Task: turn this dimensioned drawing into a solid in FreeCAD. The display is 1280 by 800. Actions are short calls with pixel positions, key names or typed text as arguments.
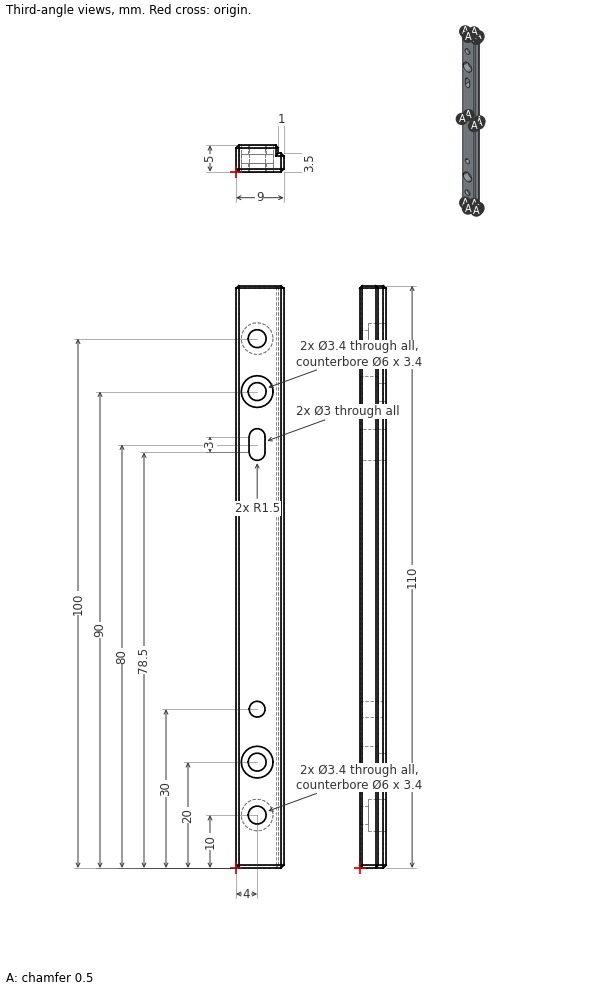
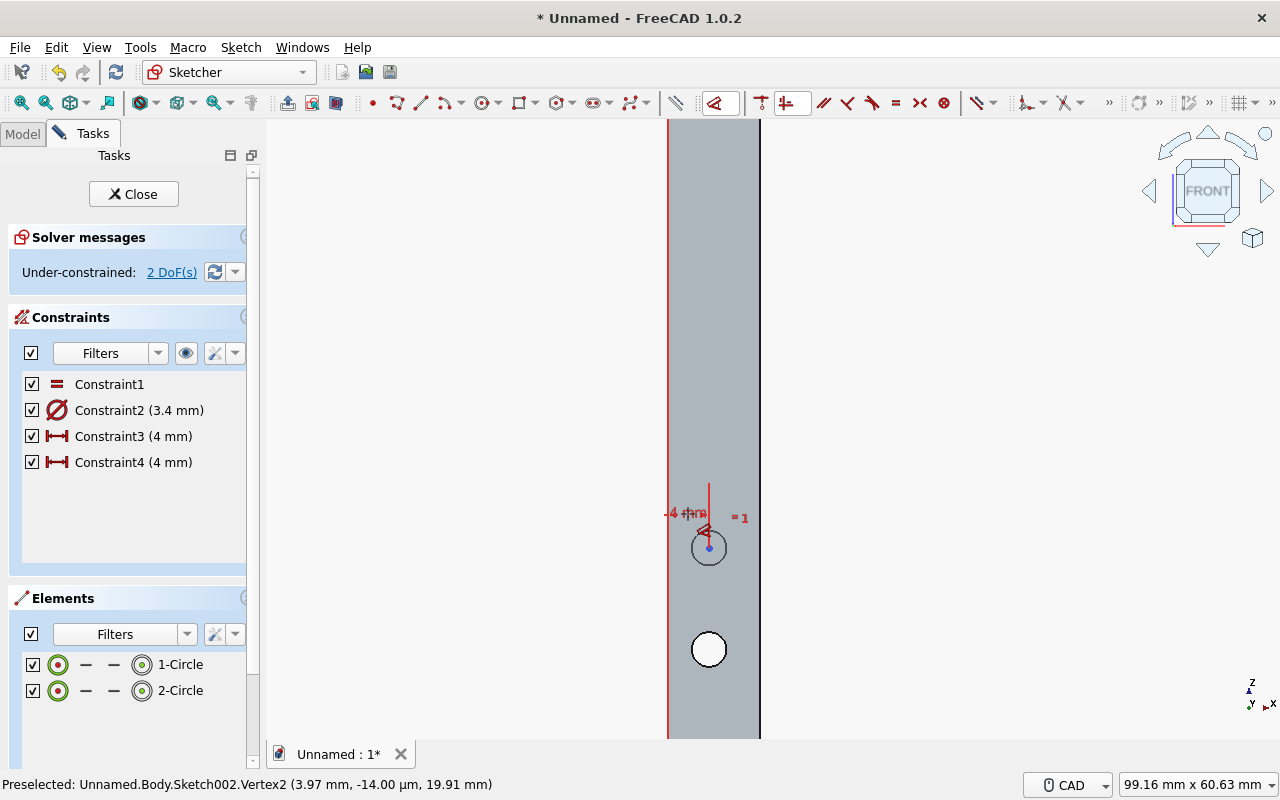
scroll(710, 548, down, 4)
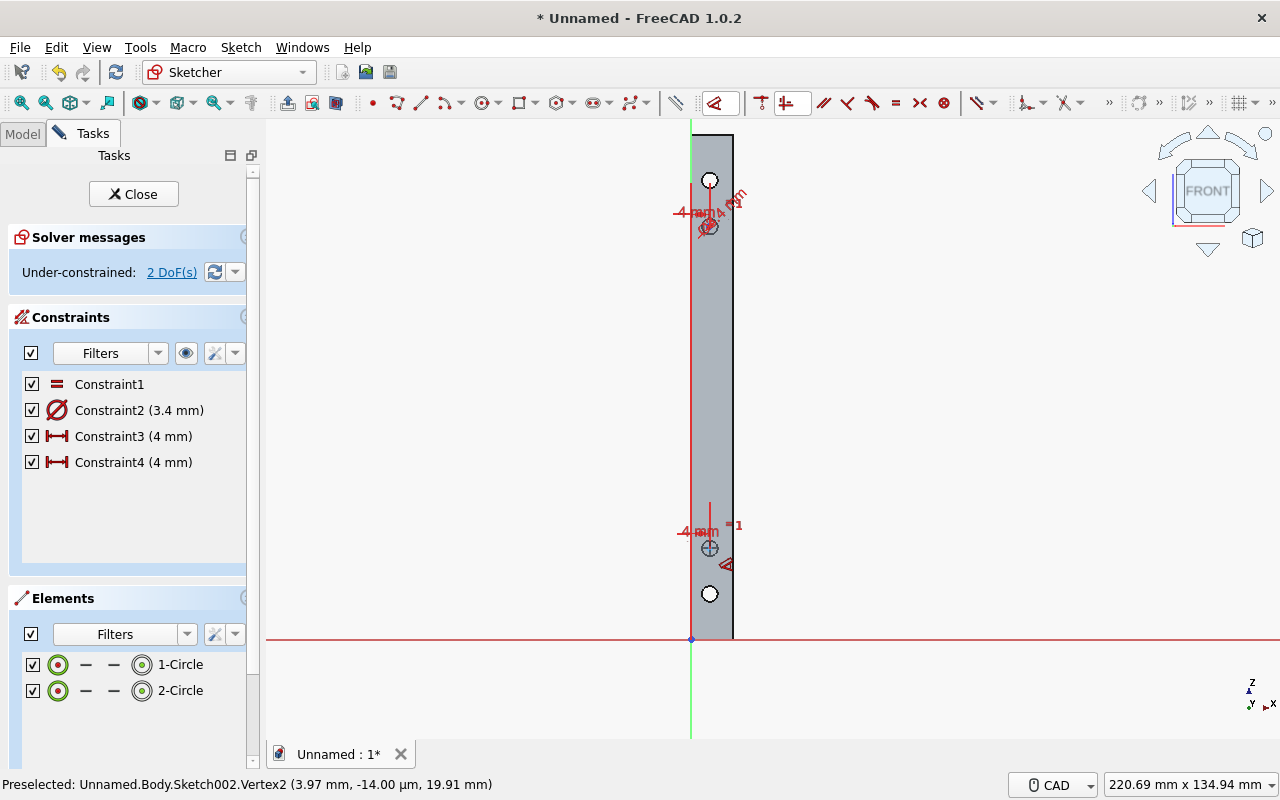
click(710, 227)
click(657, 433)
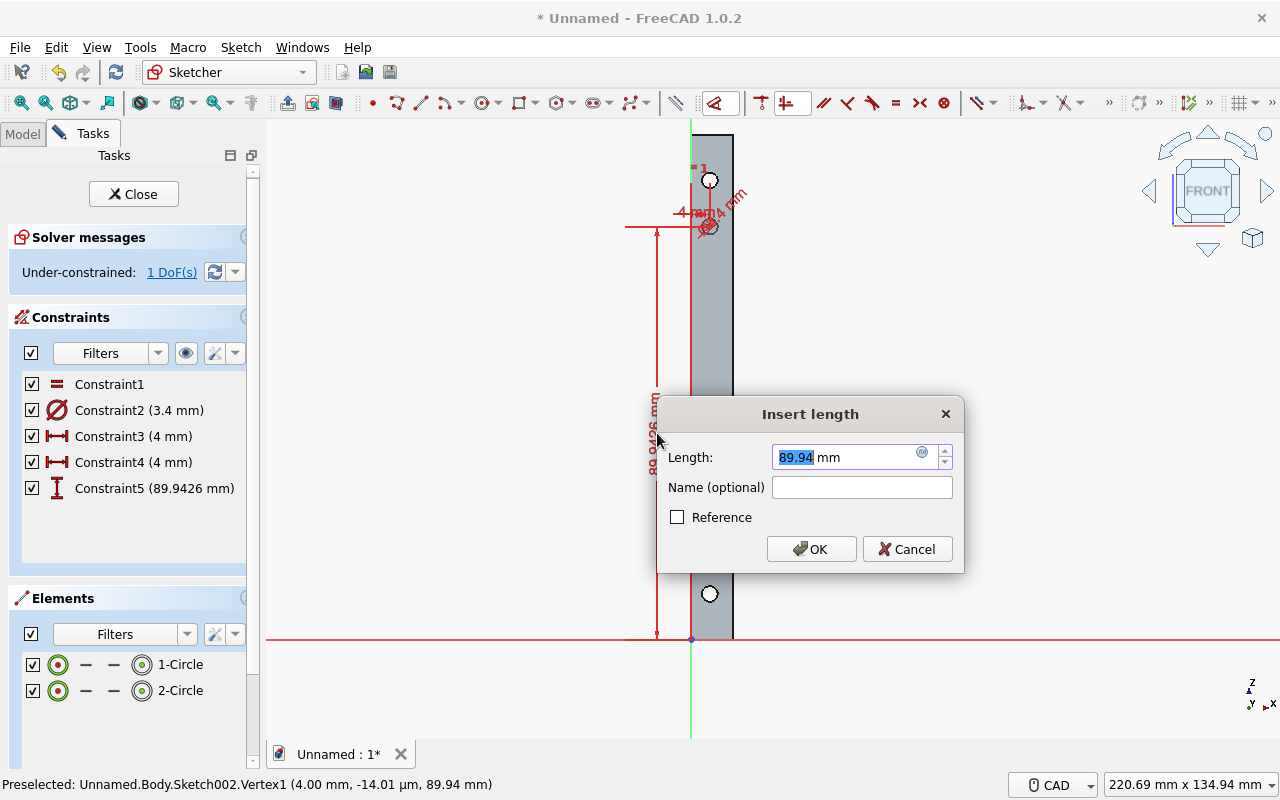
text(90)
key(Return)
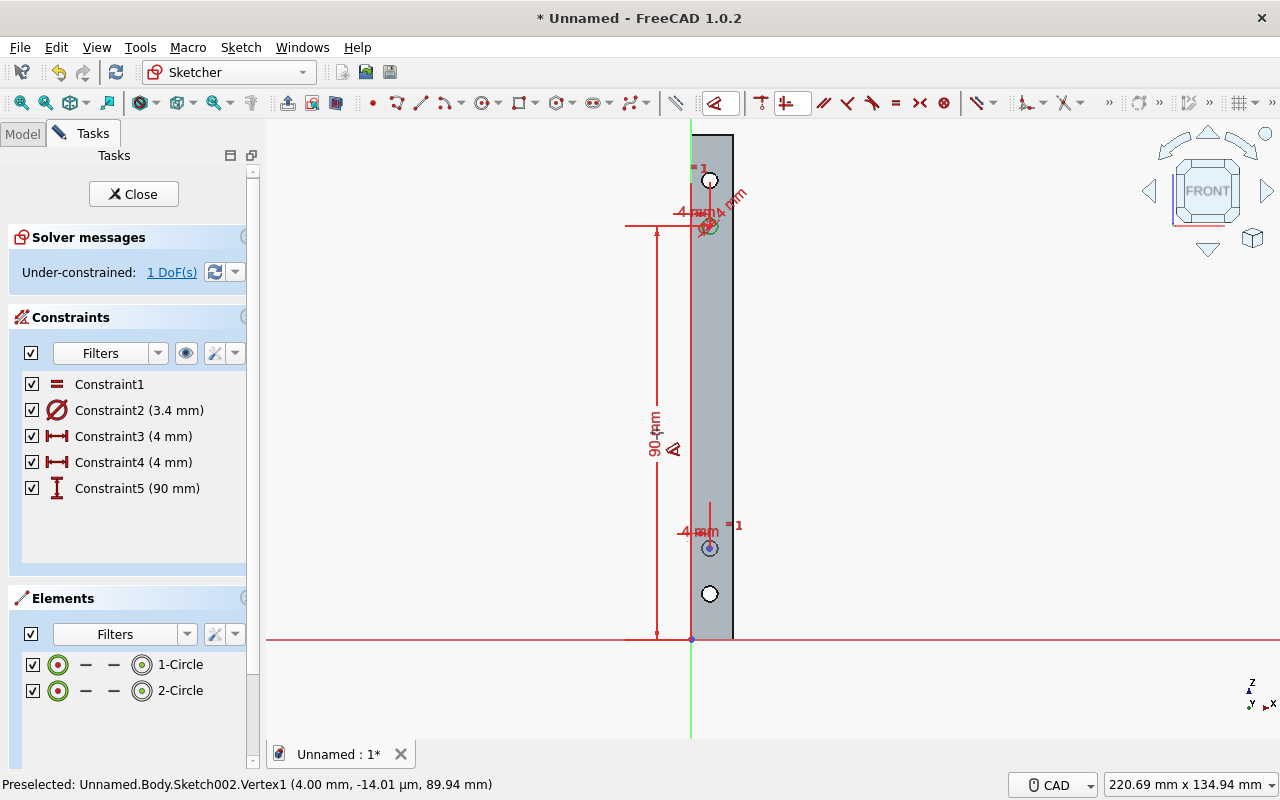
click(710, 548)
click(657, 594)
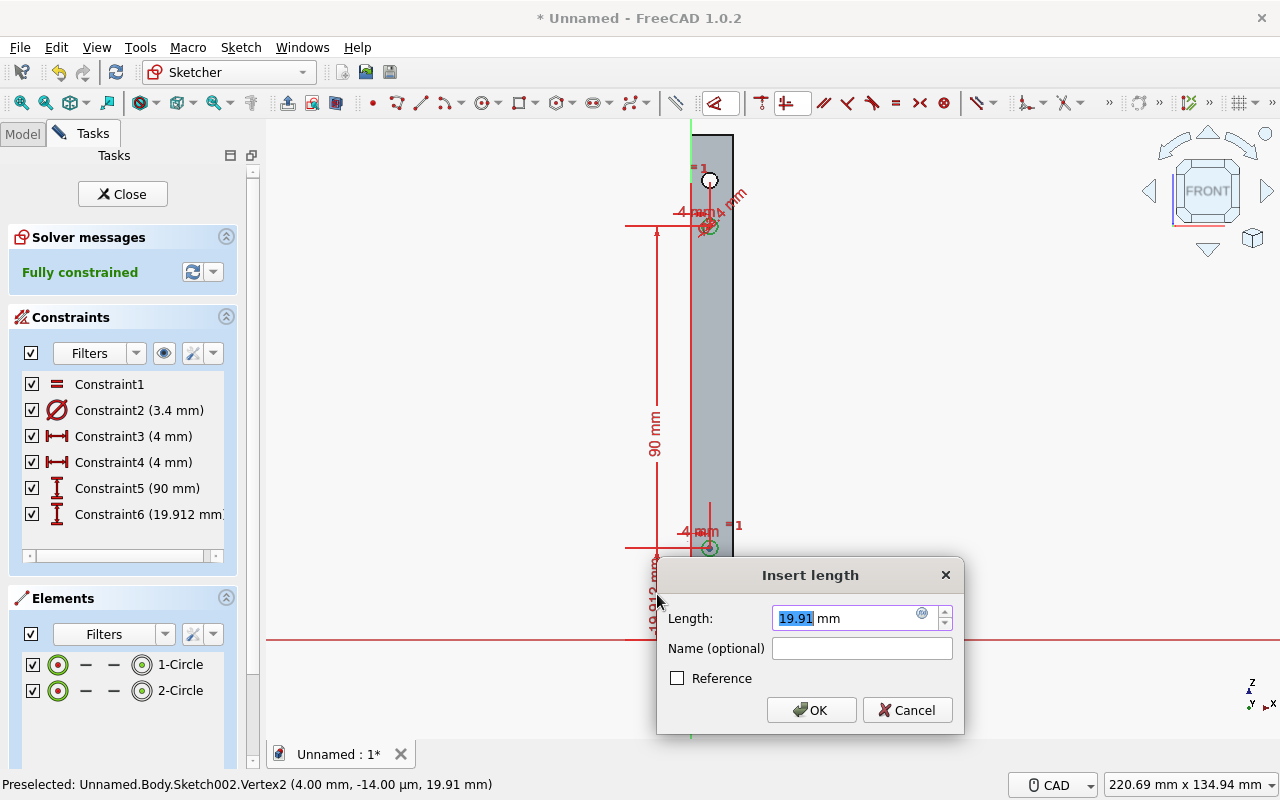
text(20)
key(Return)
key(Escape)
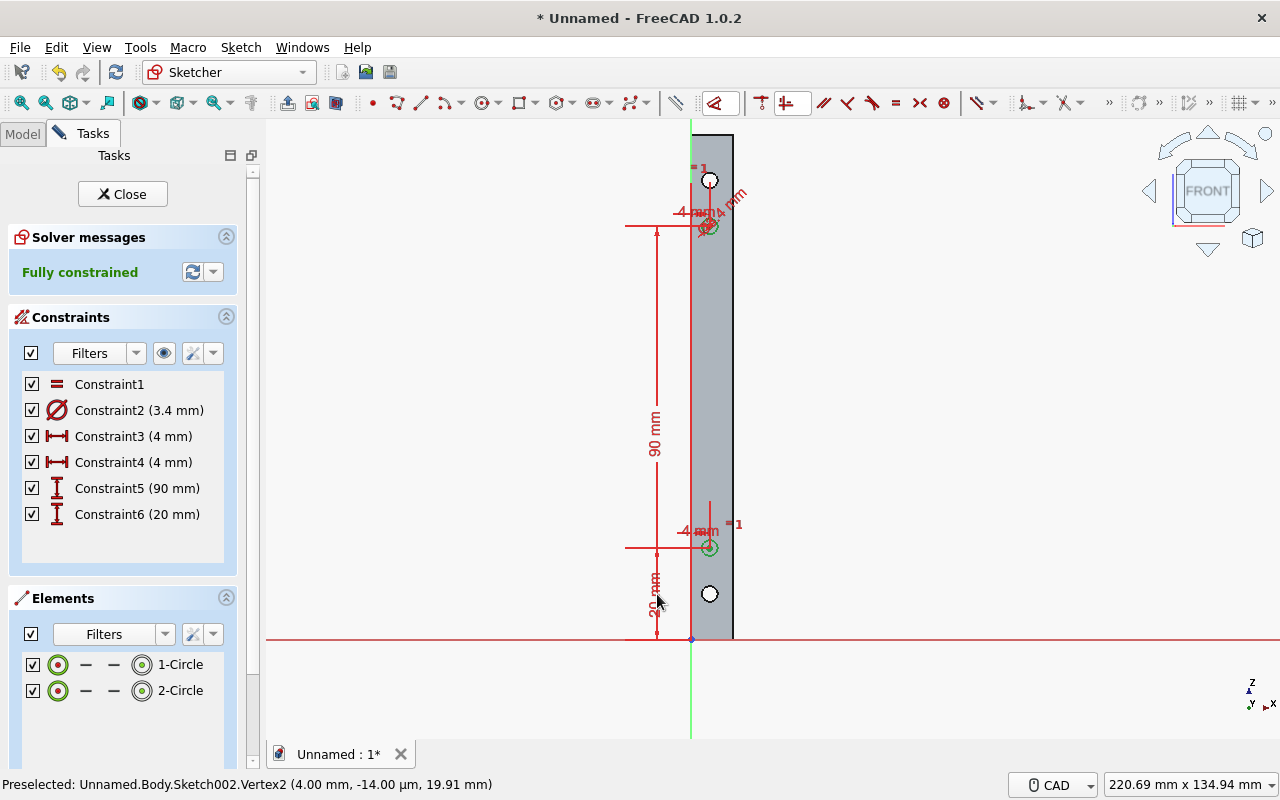
click(123, 194)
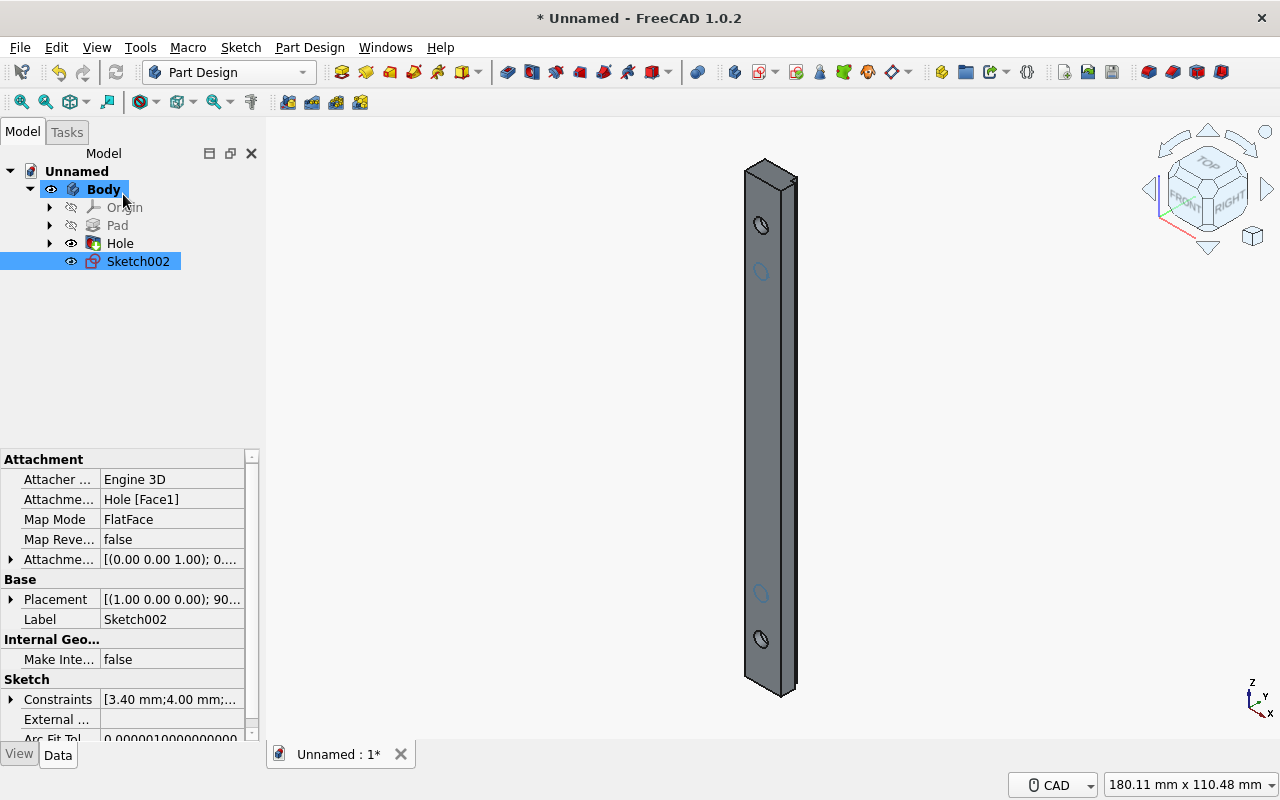
click(532, 72)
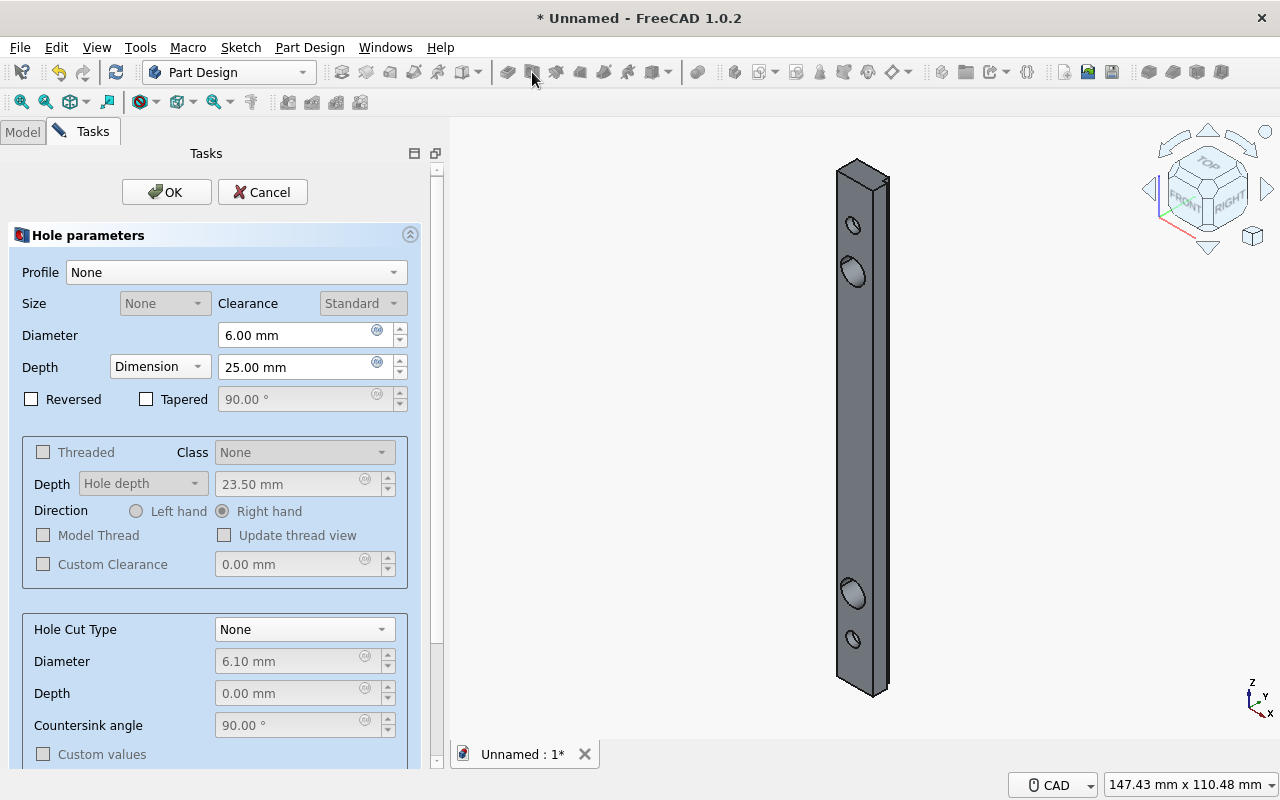
triple_click(305, 335)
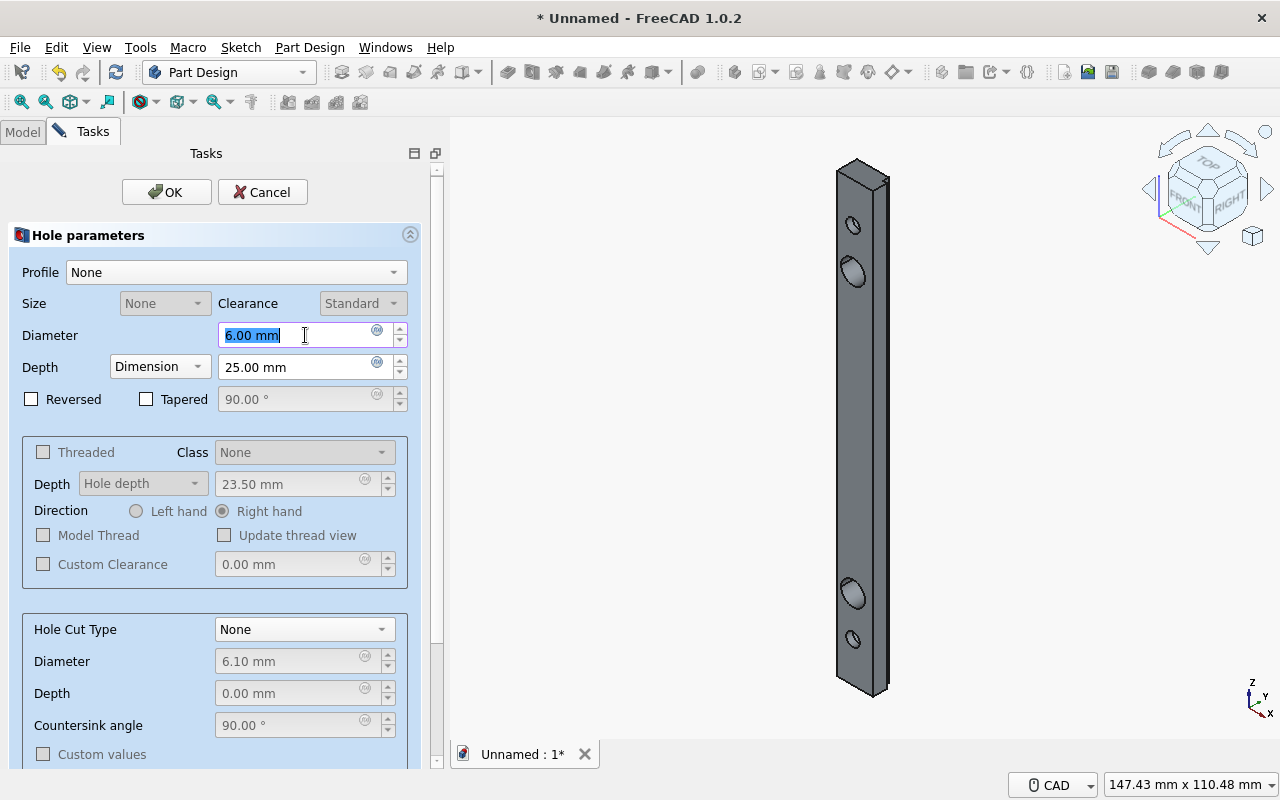
text(3.4)
key(Tab)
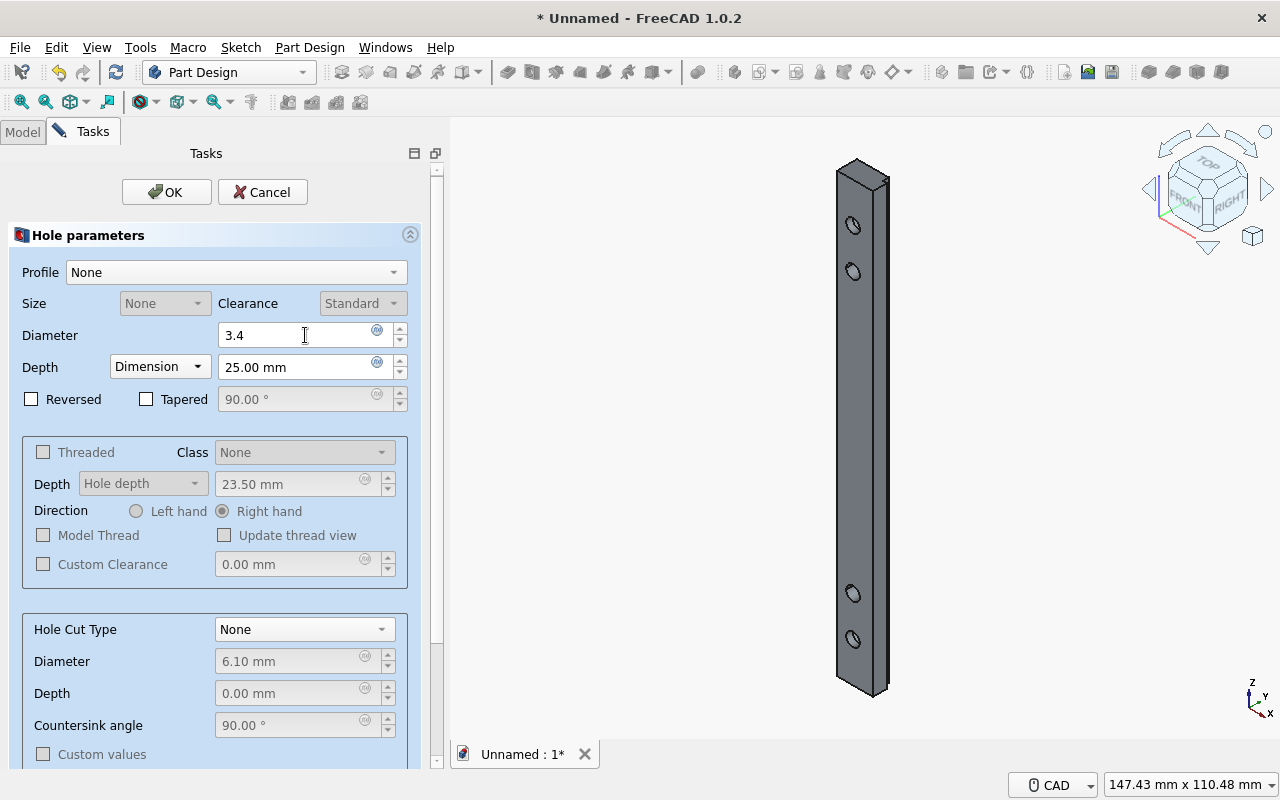
click(161, 366)